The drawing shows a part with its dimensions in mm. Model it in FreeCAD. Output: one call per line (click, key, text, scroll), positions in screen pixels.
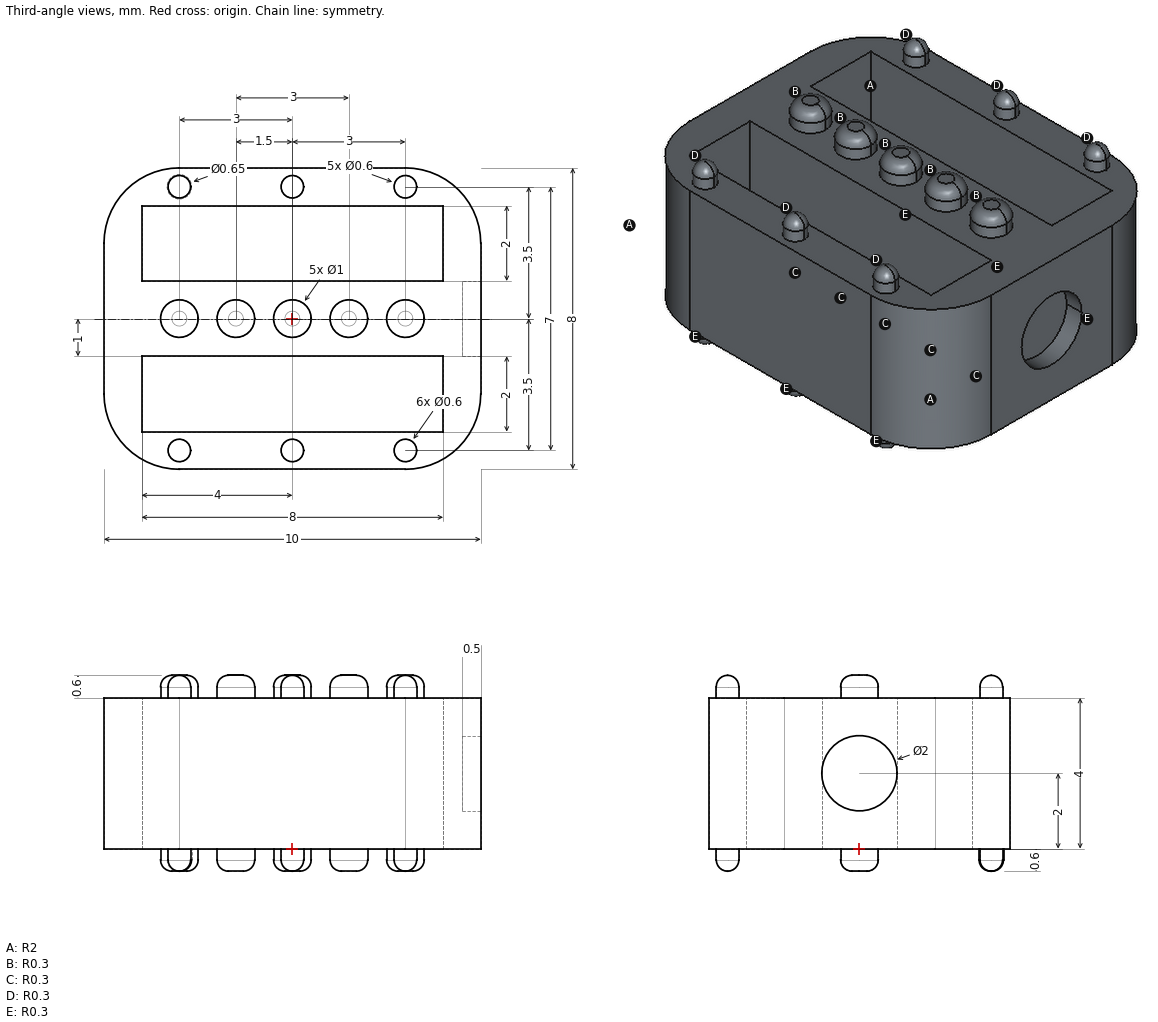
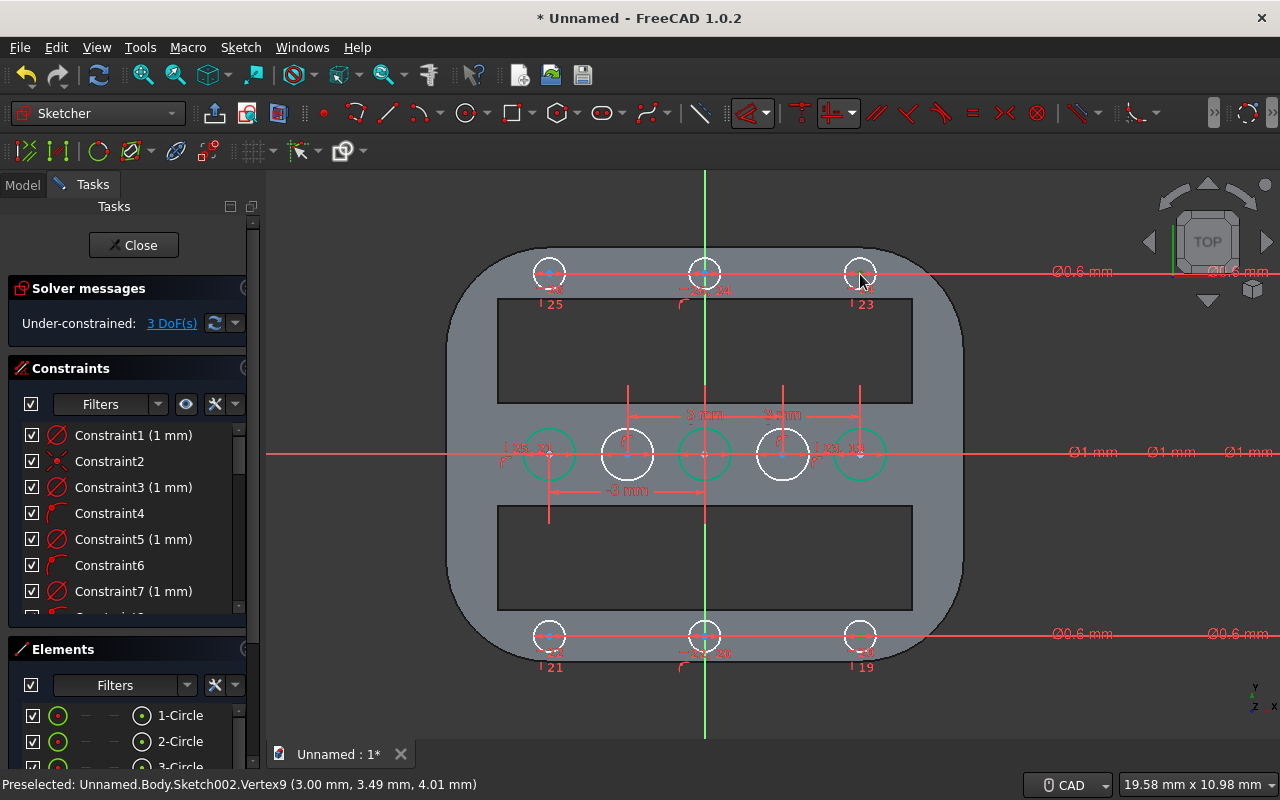
click(768, 114)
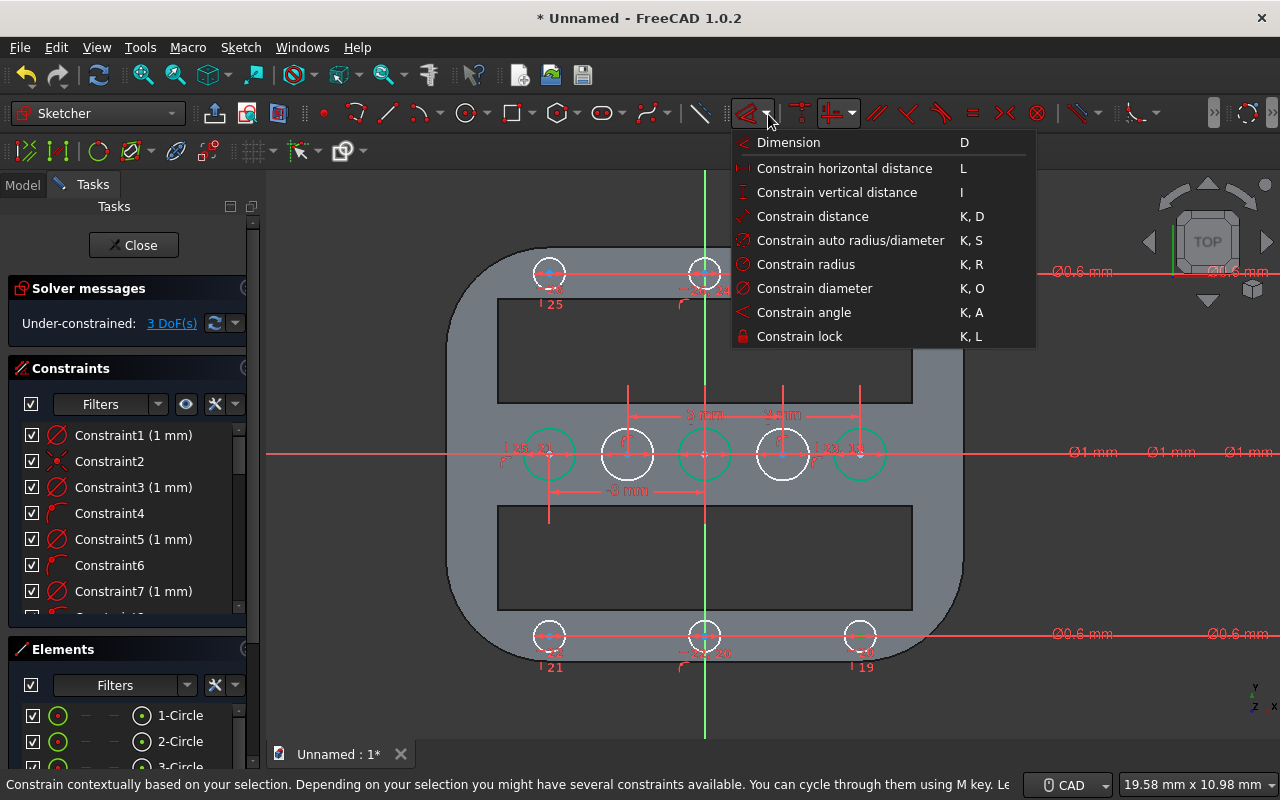
click(884, 192)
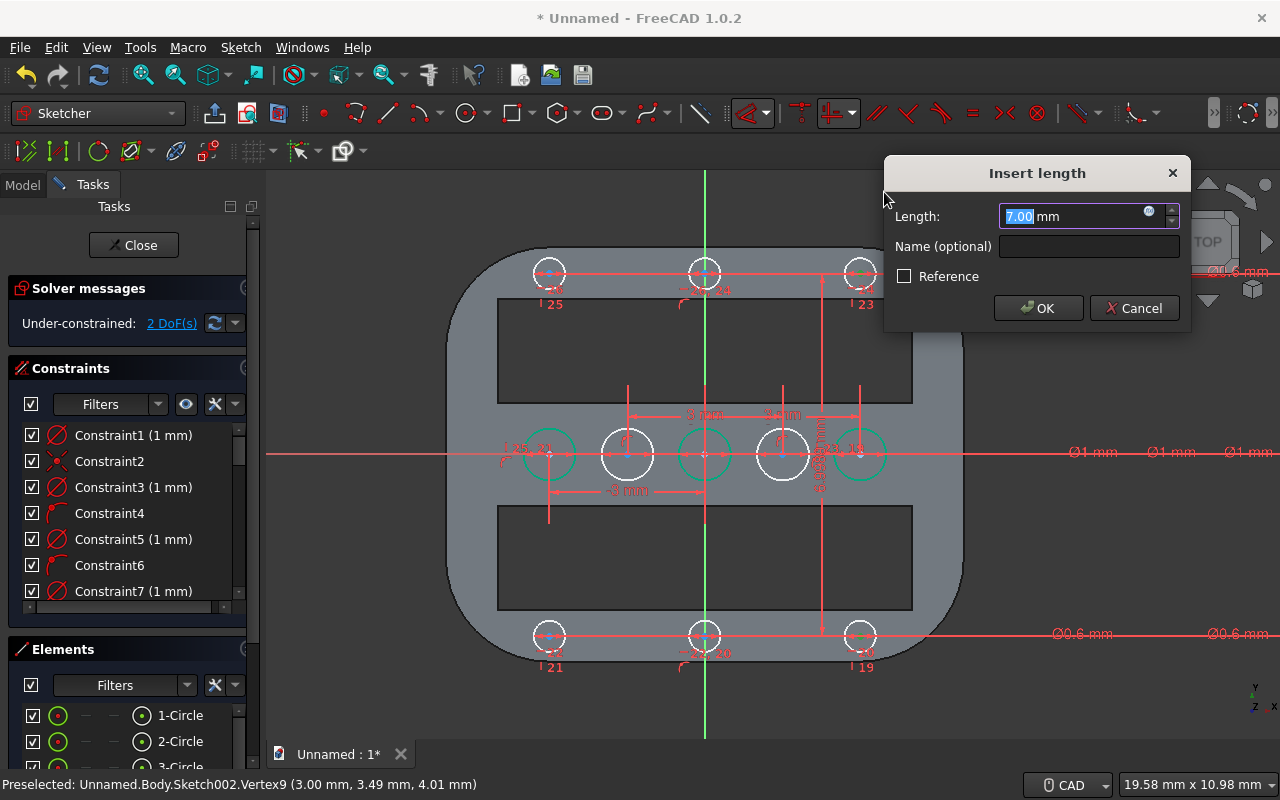
text(7)
key(Return)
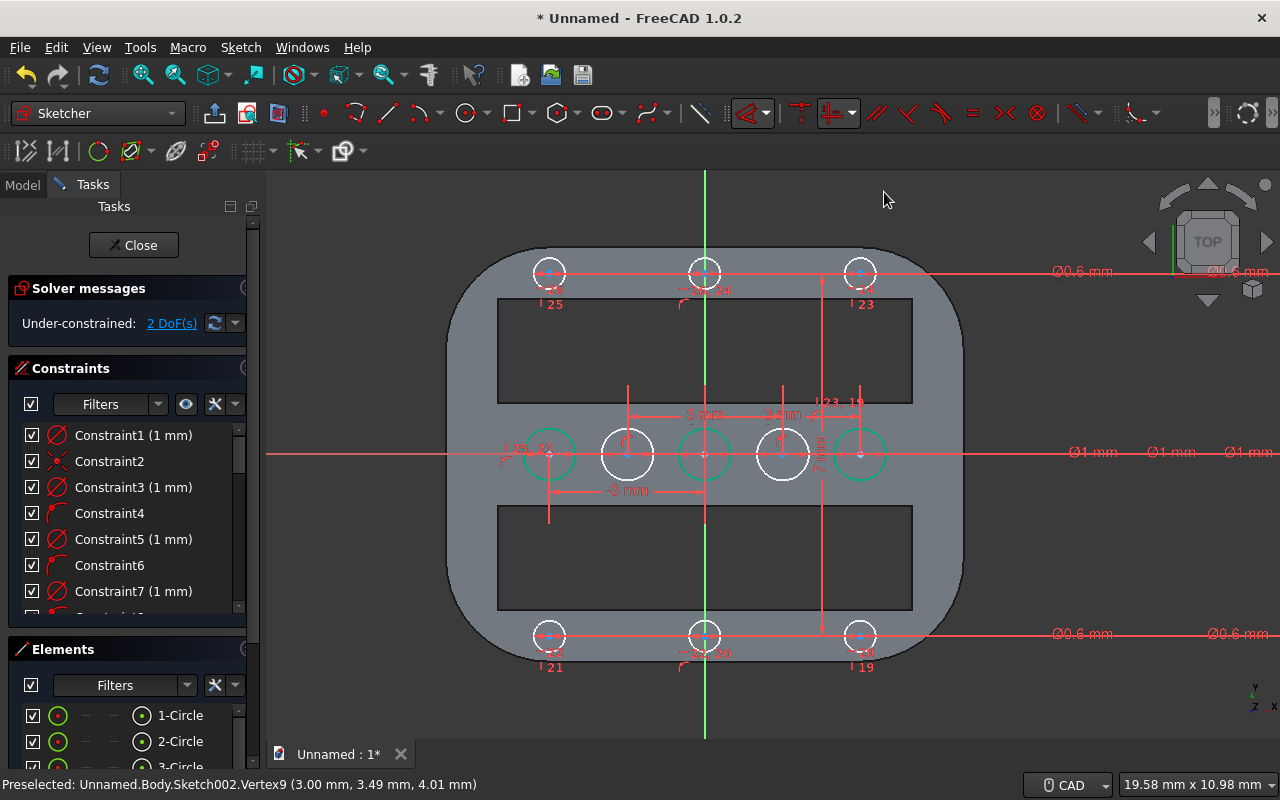
click(628, 454)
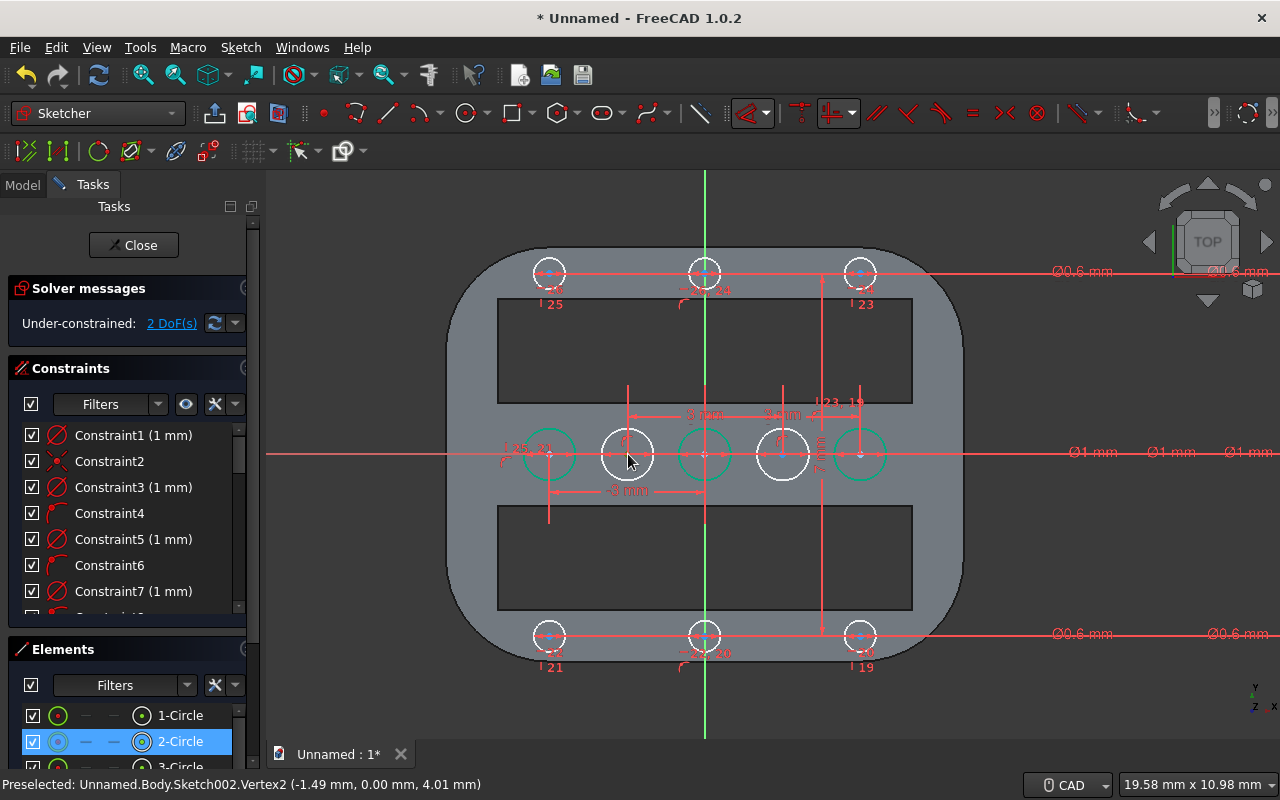
click(768, 114)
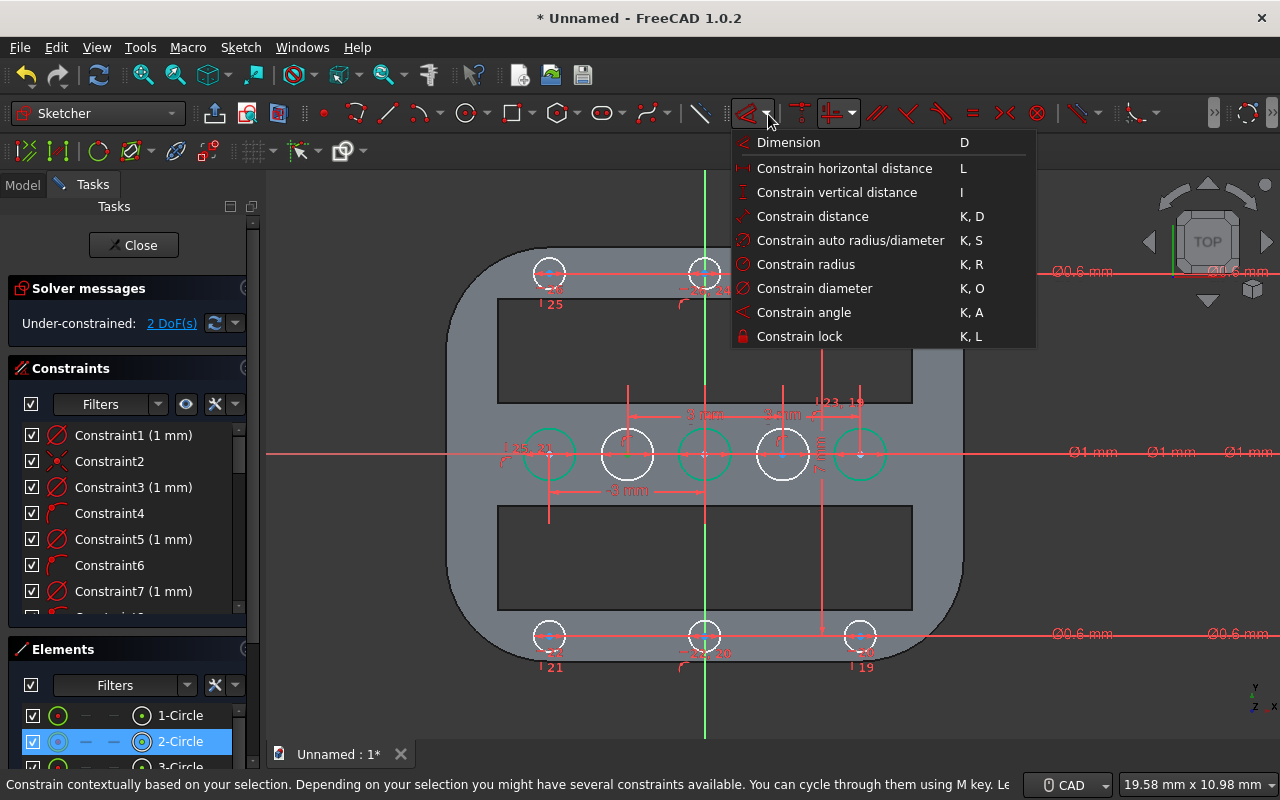
click(884, 168)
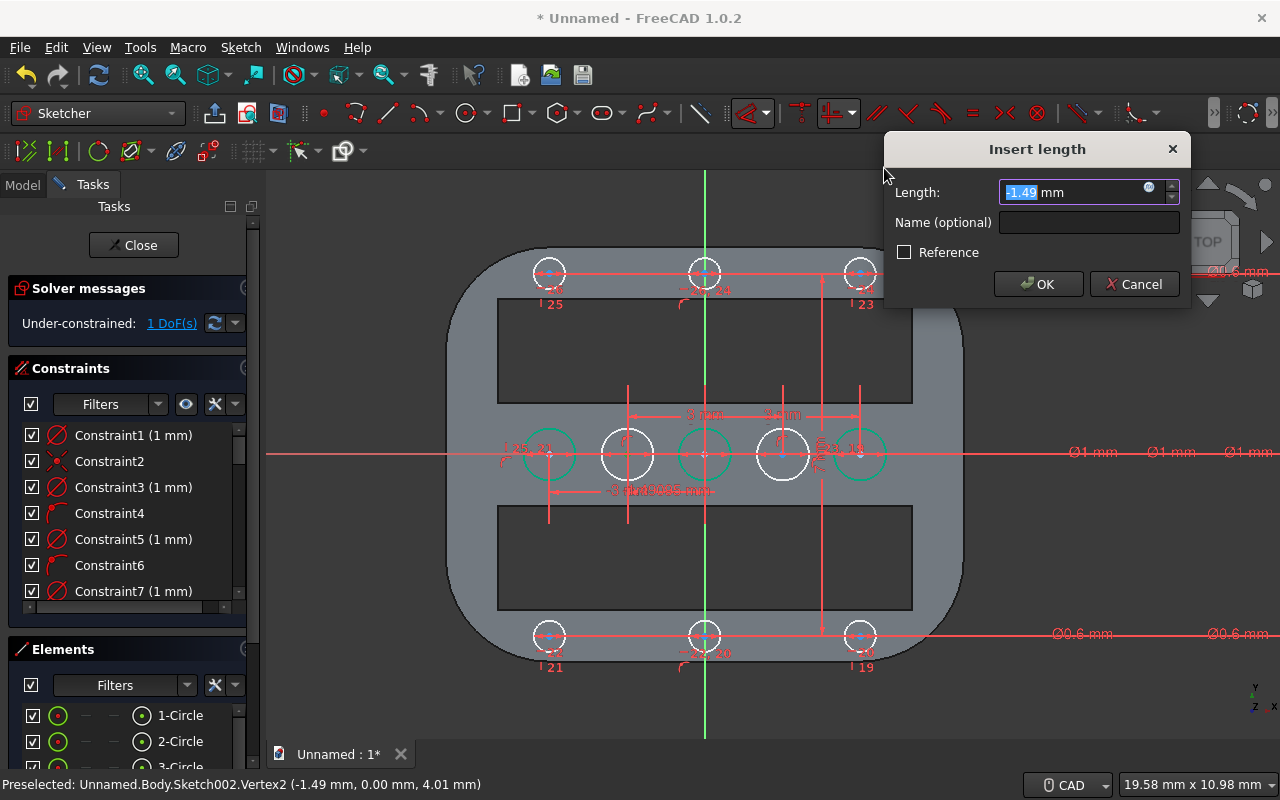
text(-1.5)
key(Return)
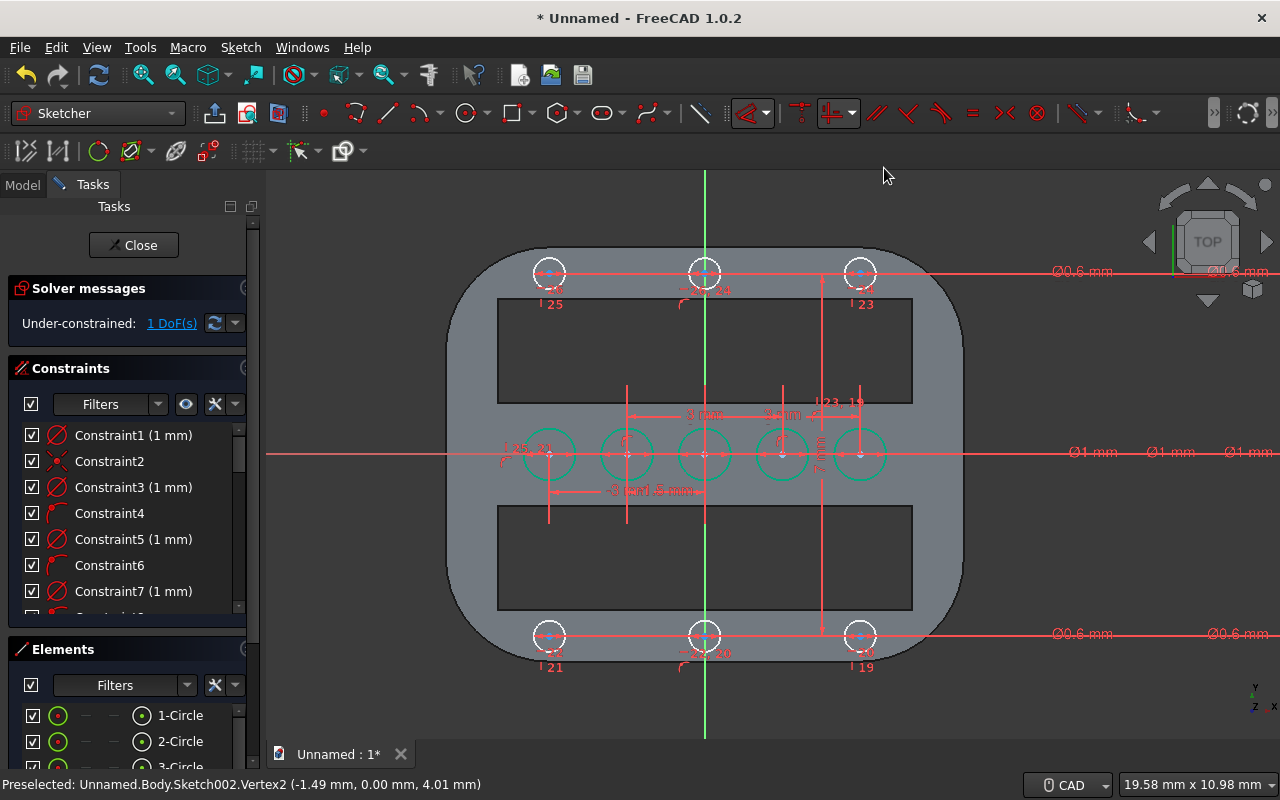
click(860, 636)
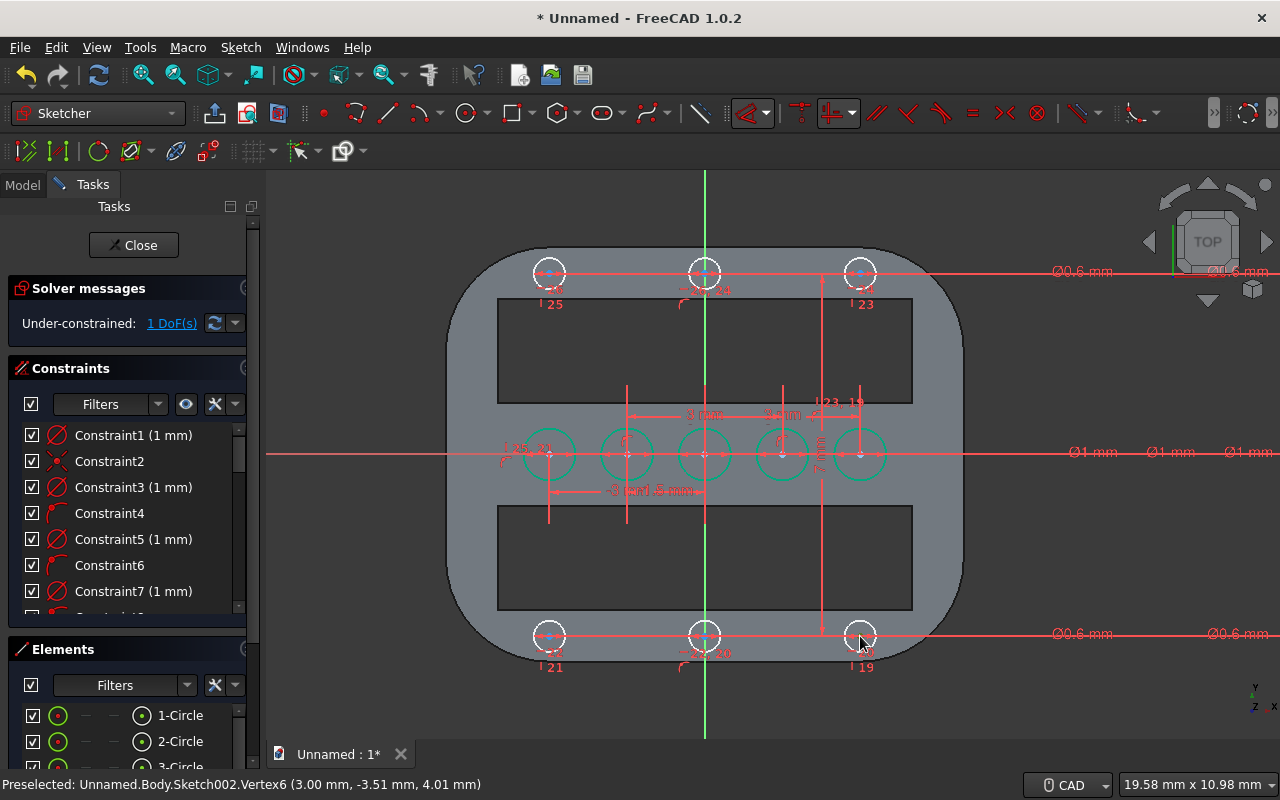
key(i)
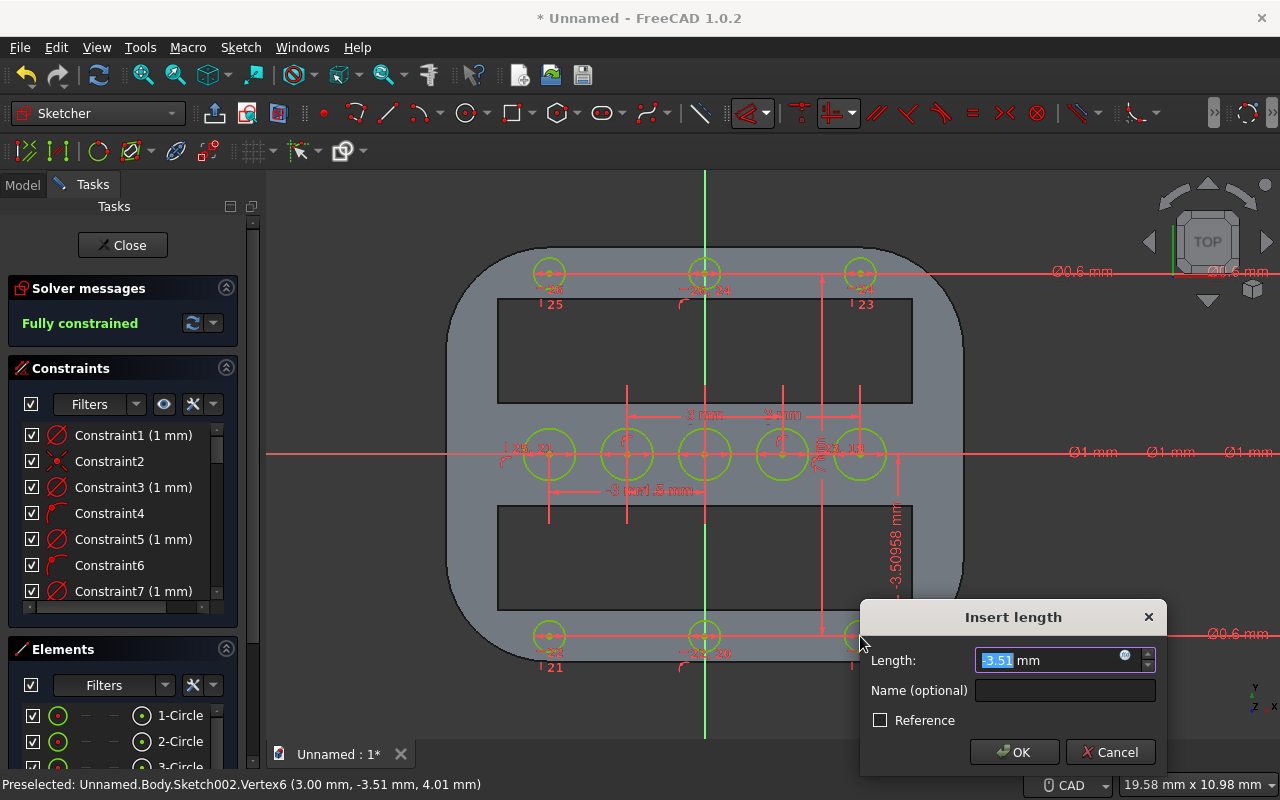
text(-3.5)
key(Return)